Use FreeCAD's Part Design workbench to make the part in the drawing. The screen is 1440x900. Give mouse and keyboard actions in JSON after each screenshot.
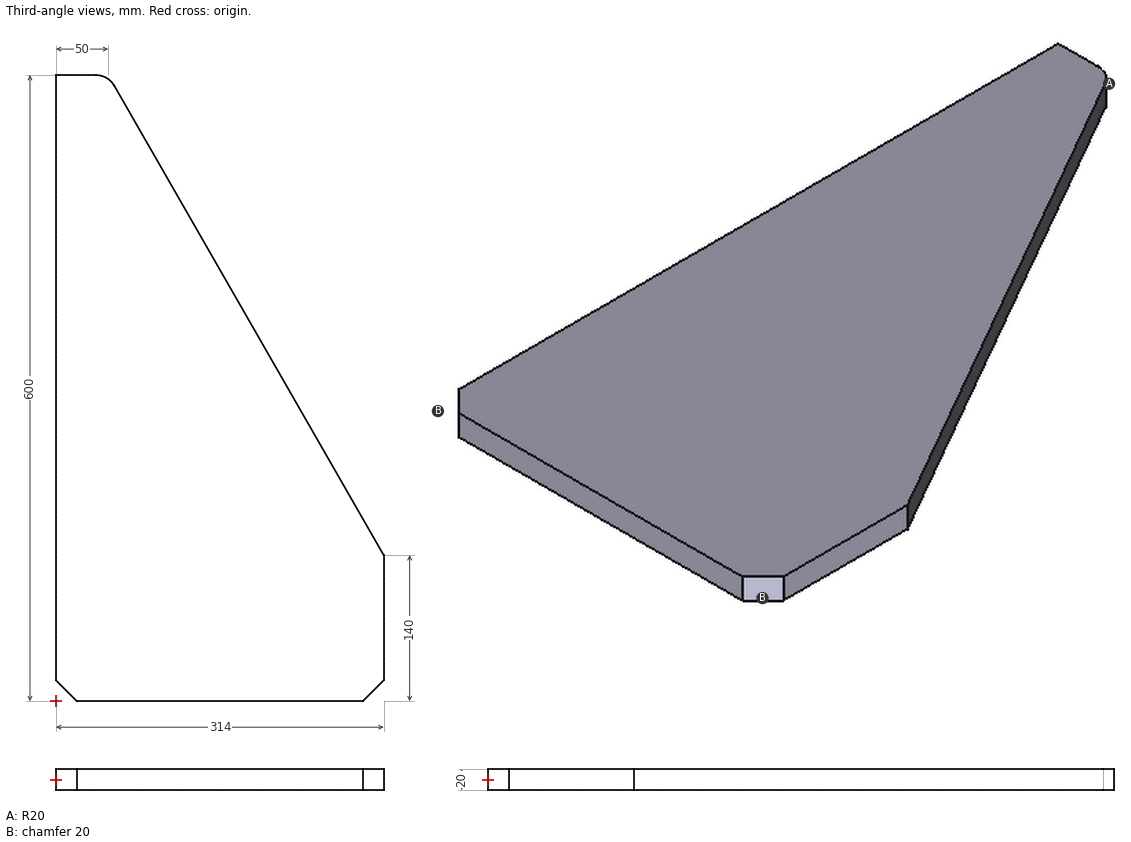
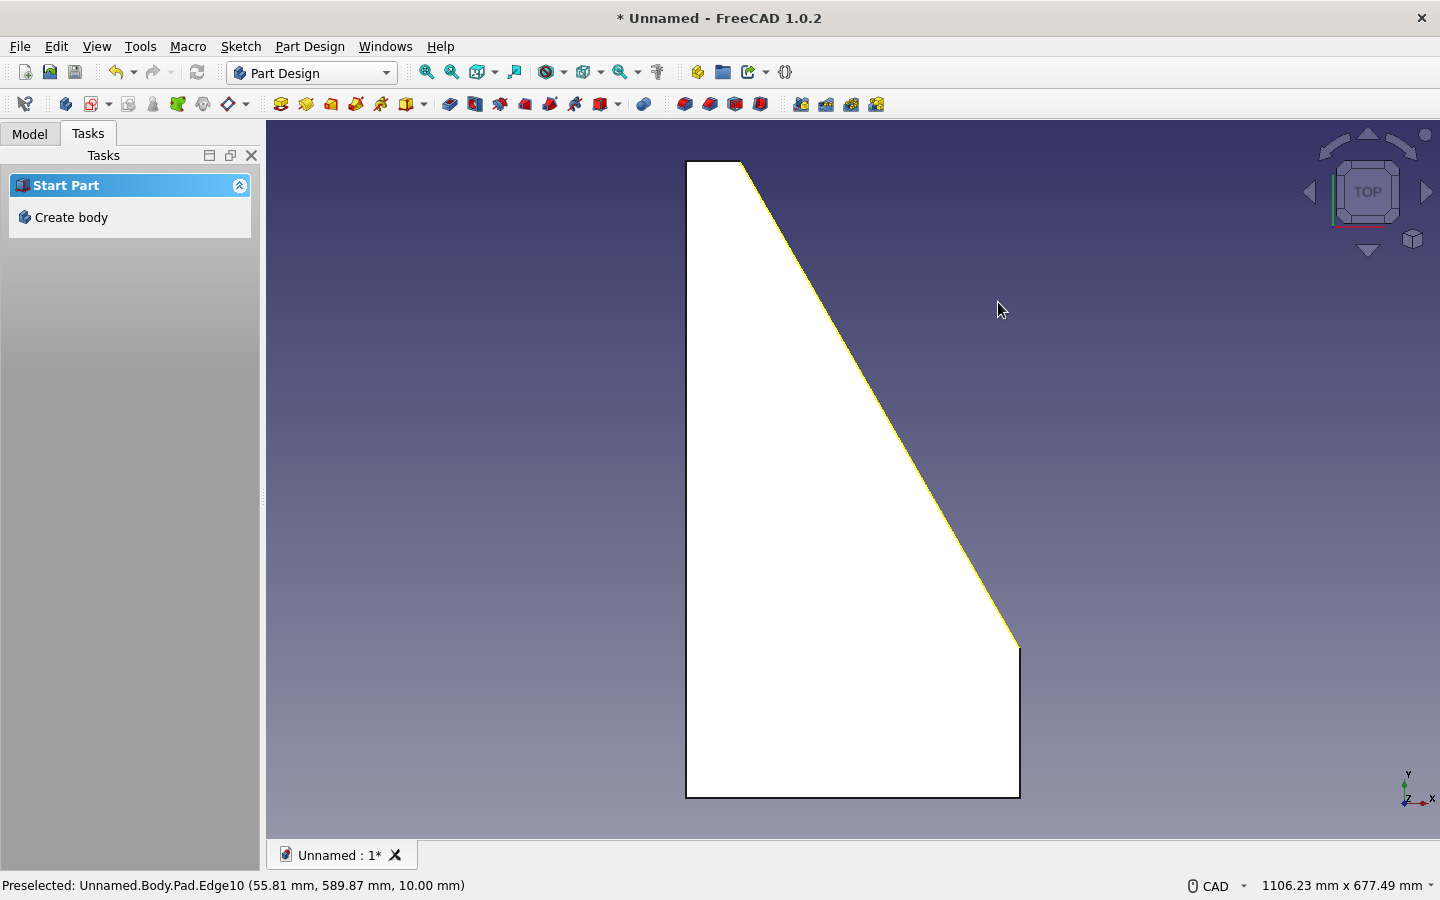
{"action": "scroll", "coordinate": [739, 160], "scroll_direction": "up", "scroll_amount": 4}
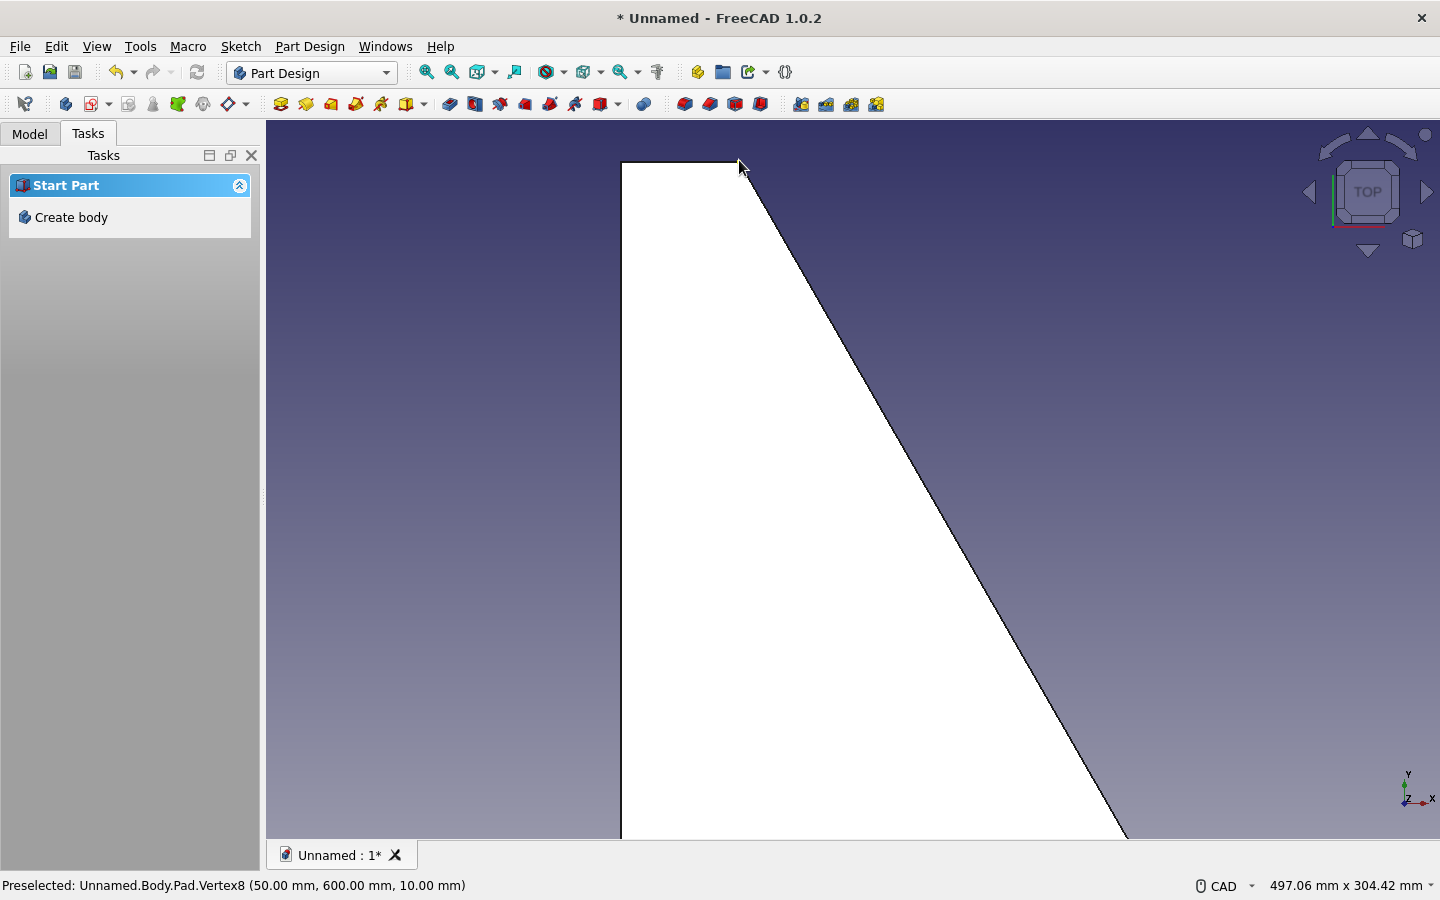
{"action": "key", "text": "v f"}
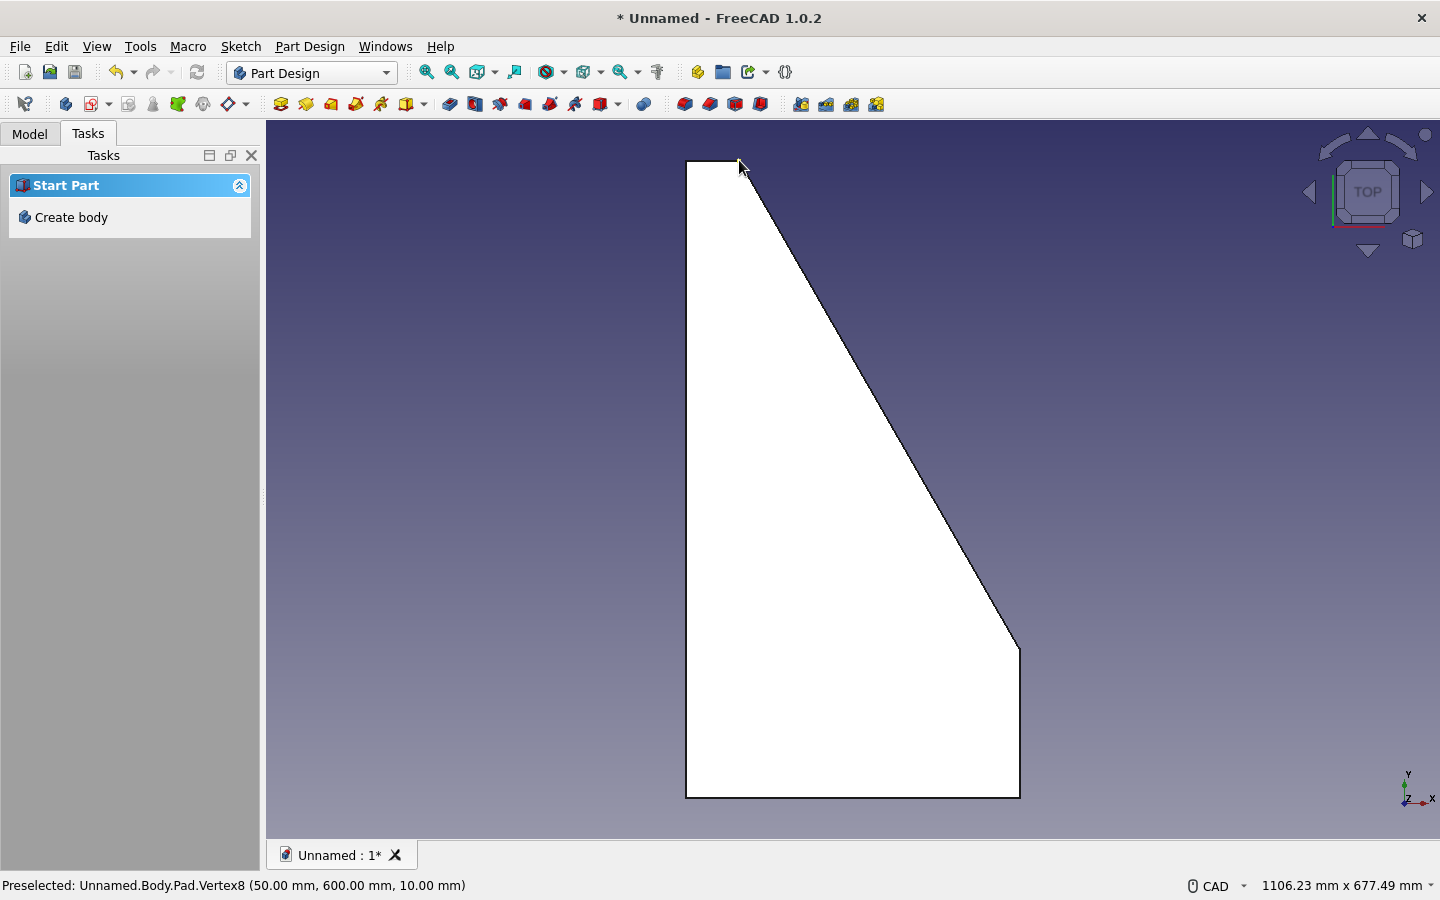
{"action": "key", "text": "1"}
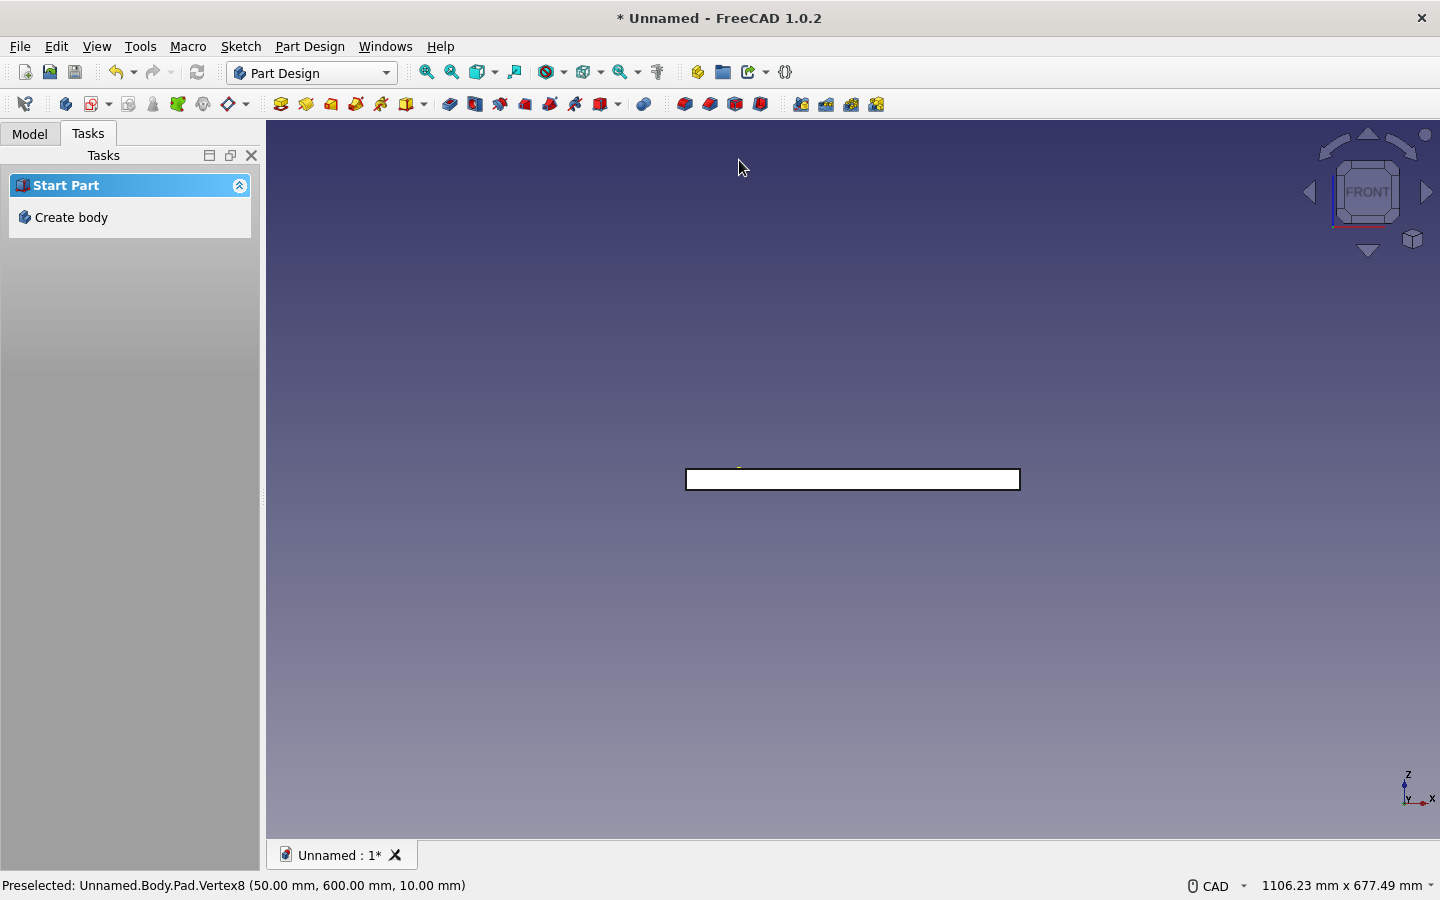
{"action": "key", "text": "v f"}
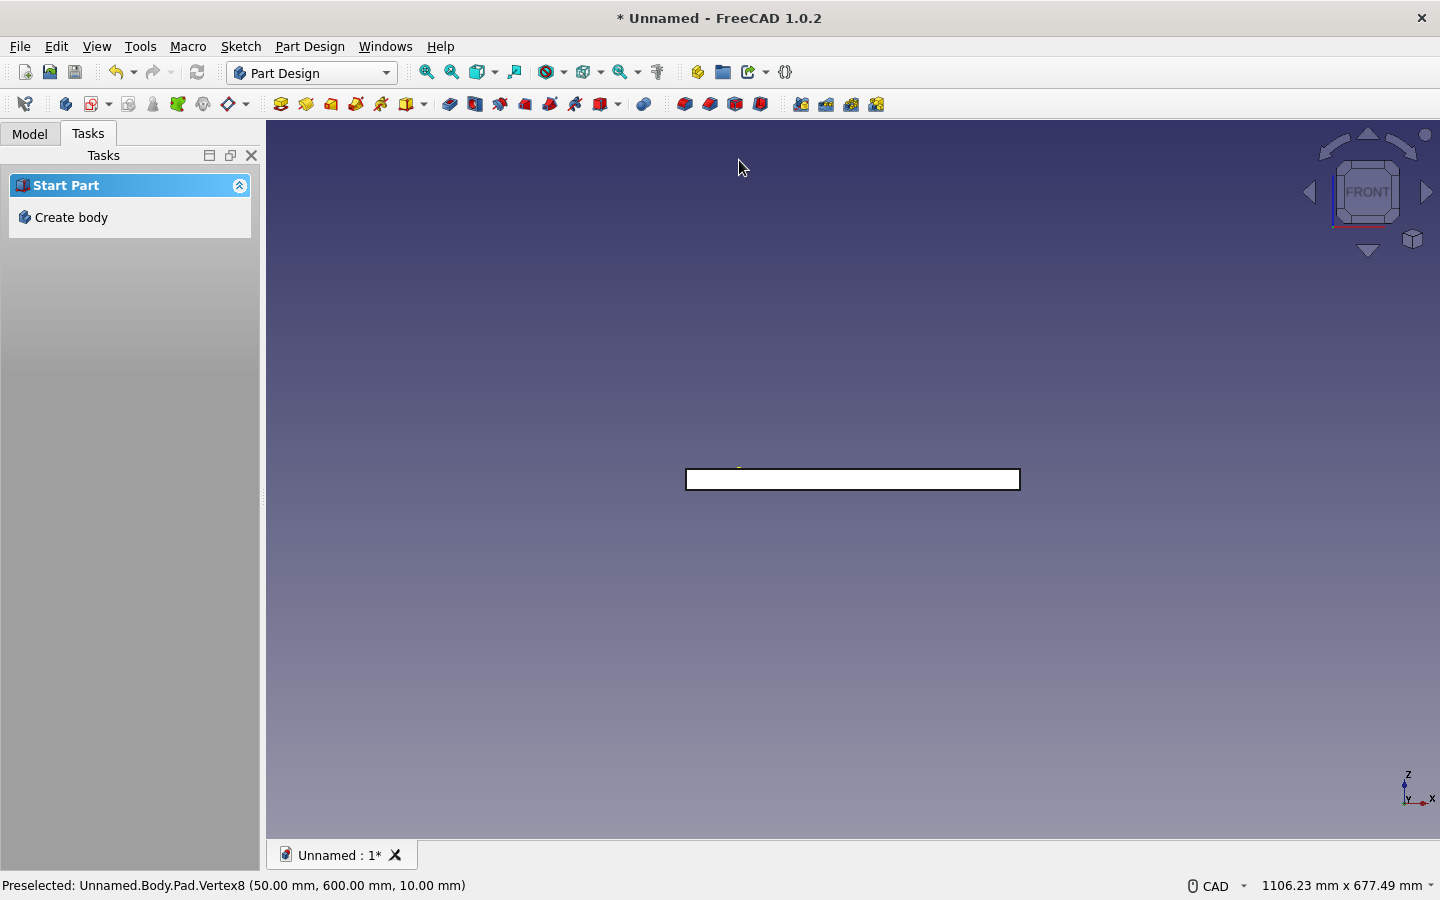
{"action": "scroll", "coordinate": [739, 479], "scroll_direction": "up", "scroll_amount": 4}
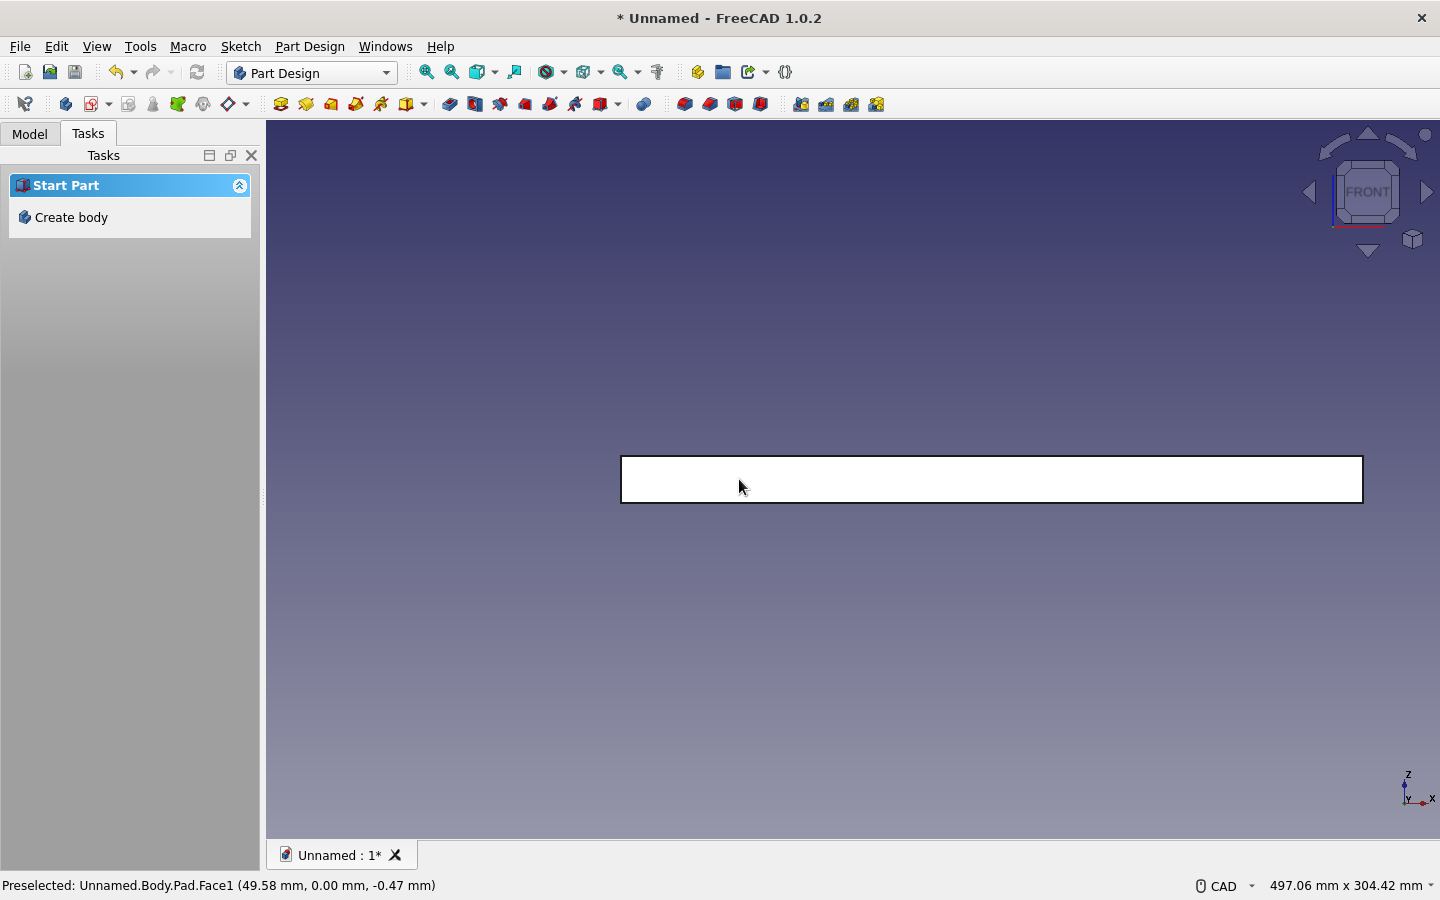
{"action": "key", "text": "v f"}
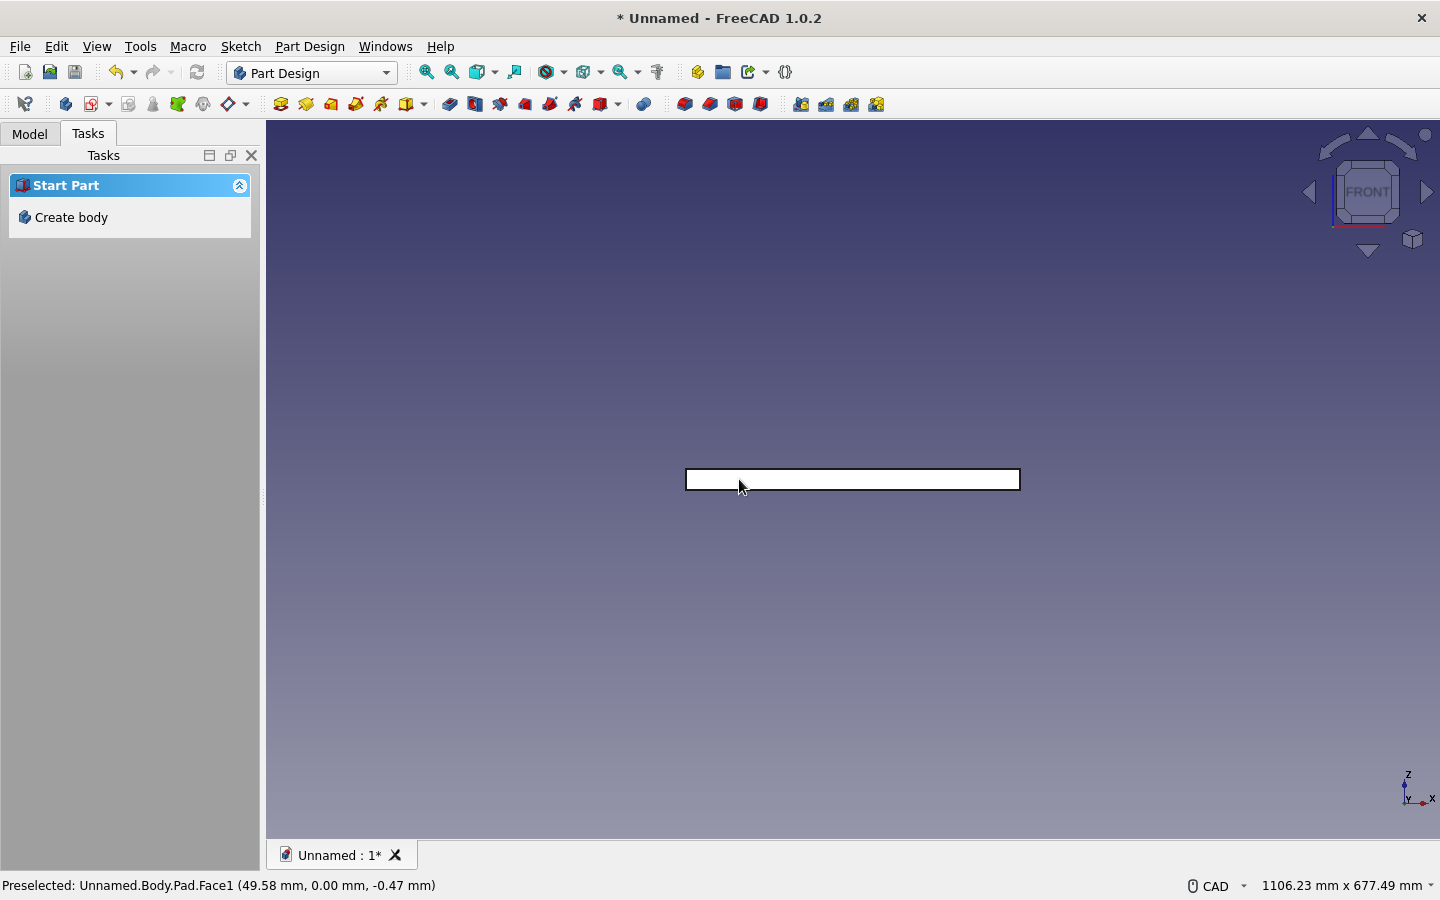
{"action": "key", "text": "3"}